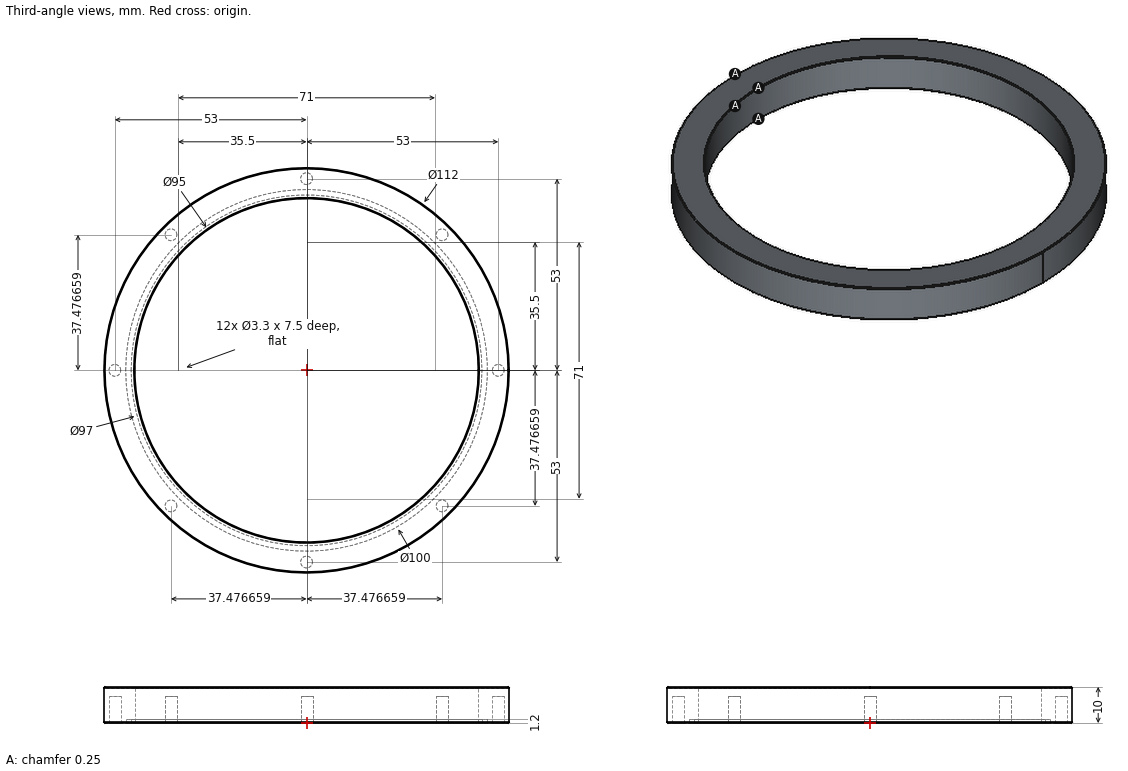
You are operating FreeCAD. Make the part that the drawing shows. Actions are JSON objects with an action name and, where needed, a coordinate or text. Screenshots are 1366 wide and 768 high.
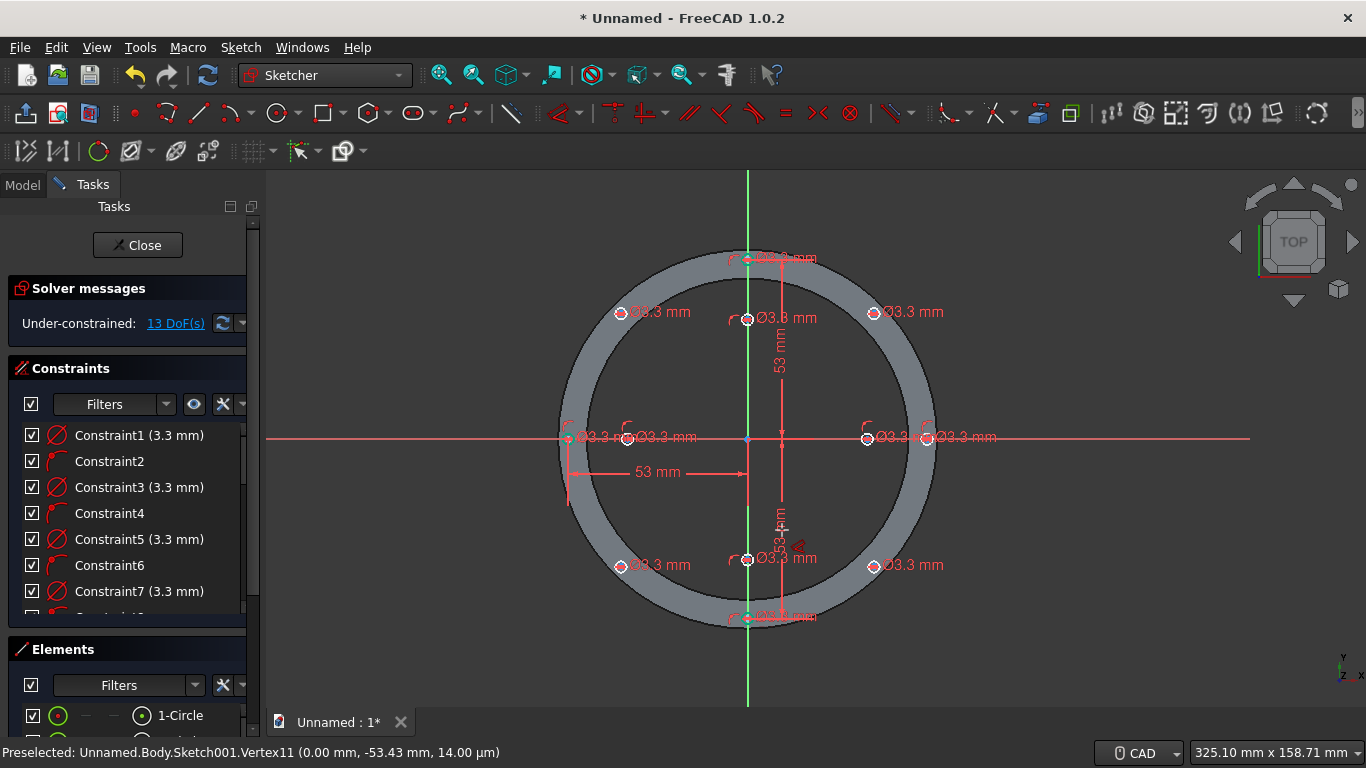
{"action": "left_click", "coordinate": [927, 439]}
{"action": "left_click", "coordinate": [837, 473]}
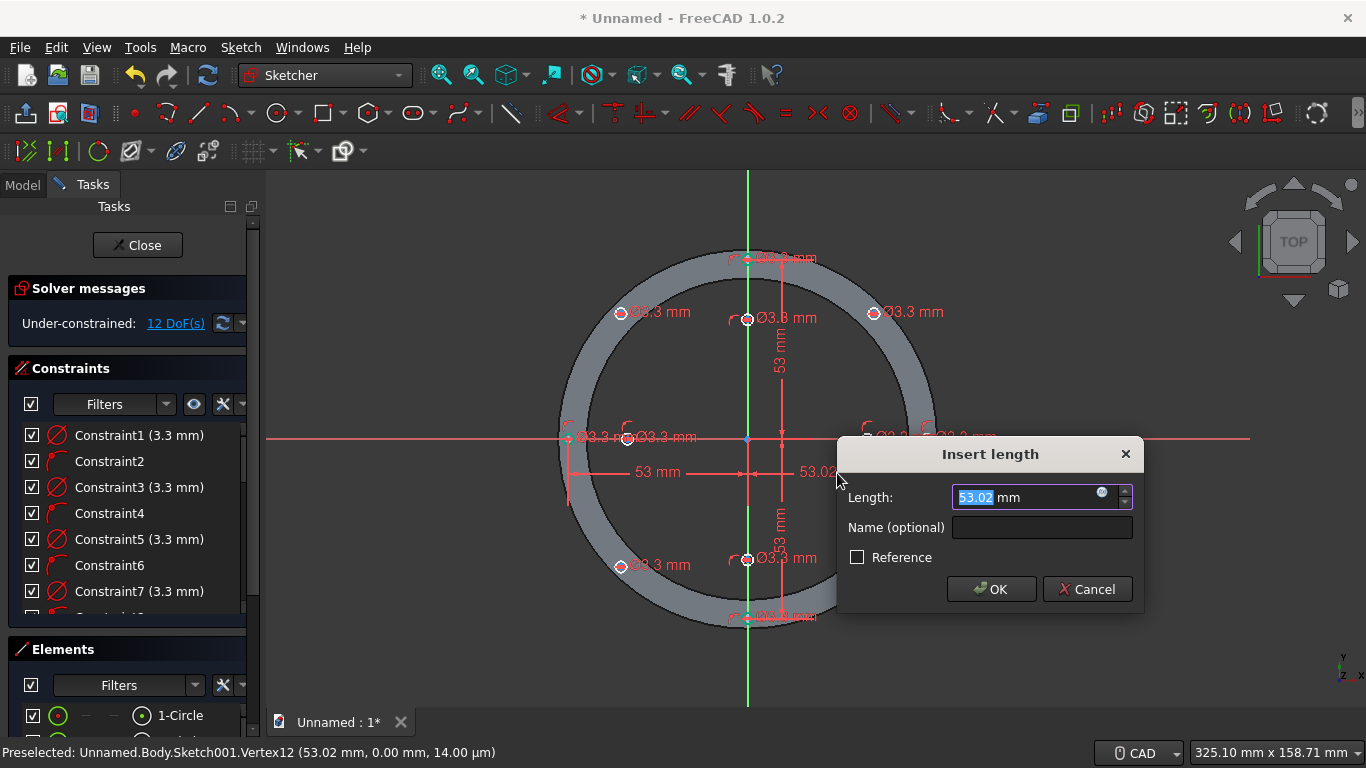
{"action": "type", "text": "53"}
{"action": "key", "text": "Return"}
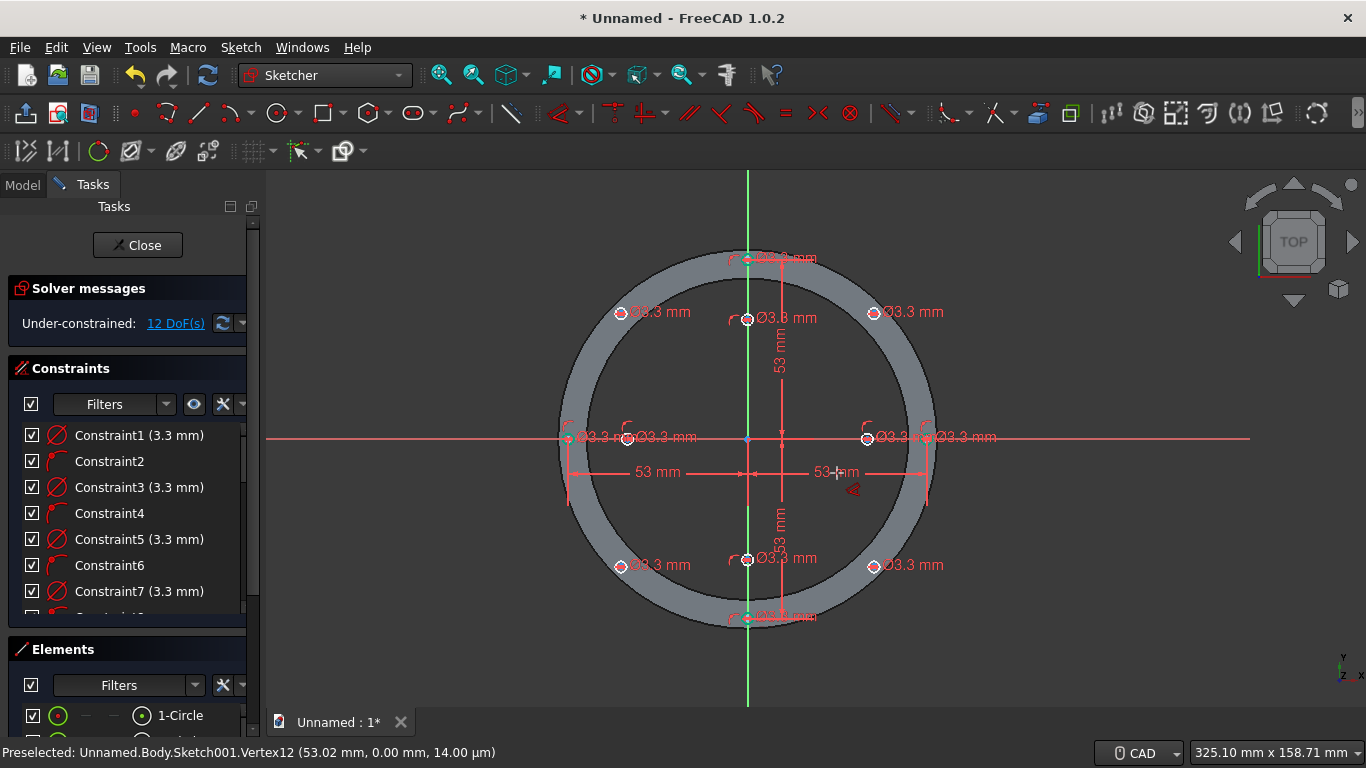
{"action": "left_click", "coordinate": [748, 320]}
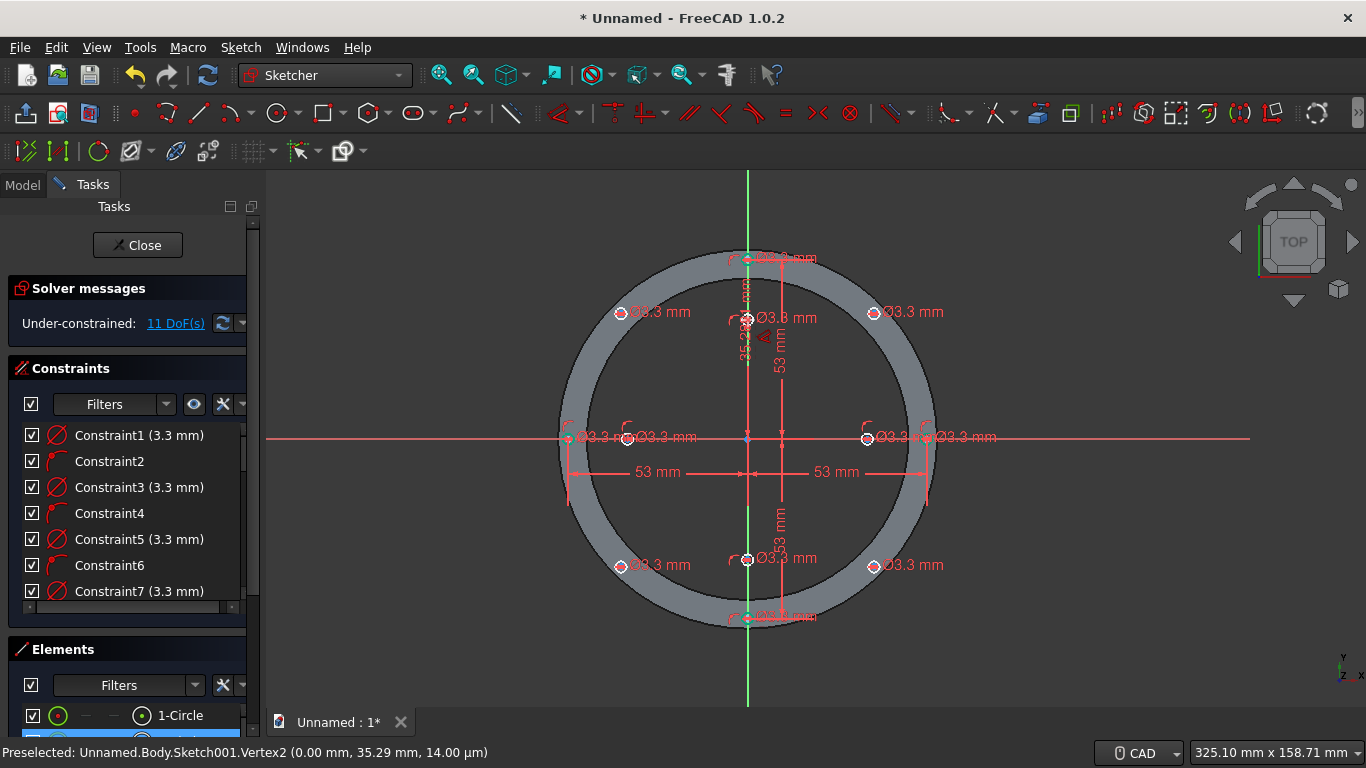
{"action": "left_click", "coordinate": [748, 560]}
{"action": "left_click", "coordinate": [782, 385]}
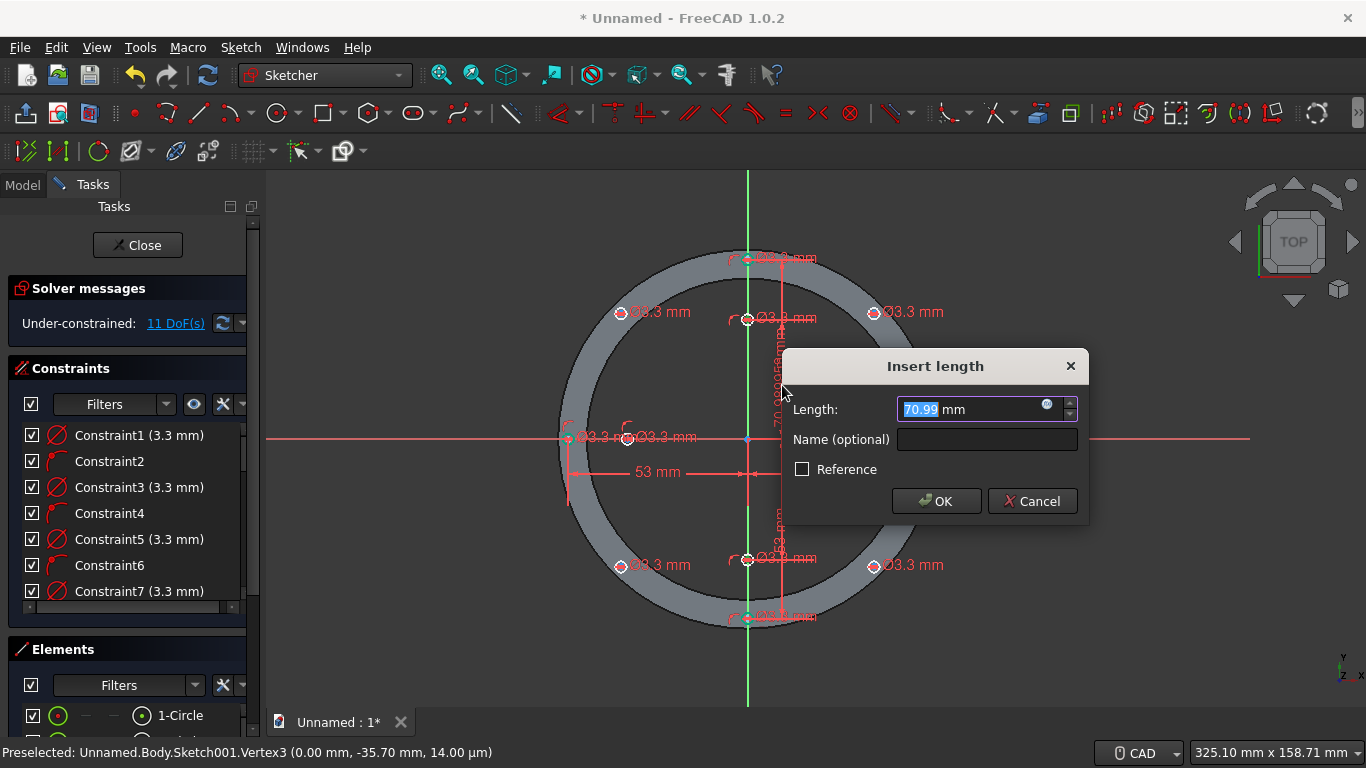
{"action": "type", "text": "71"}
{"action": "key", "text": "Return"}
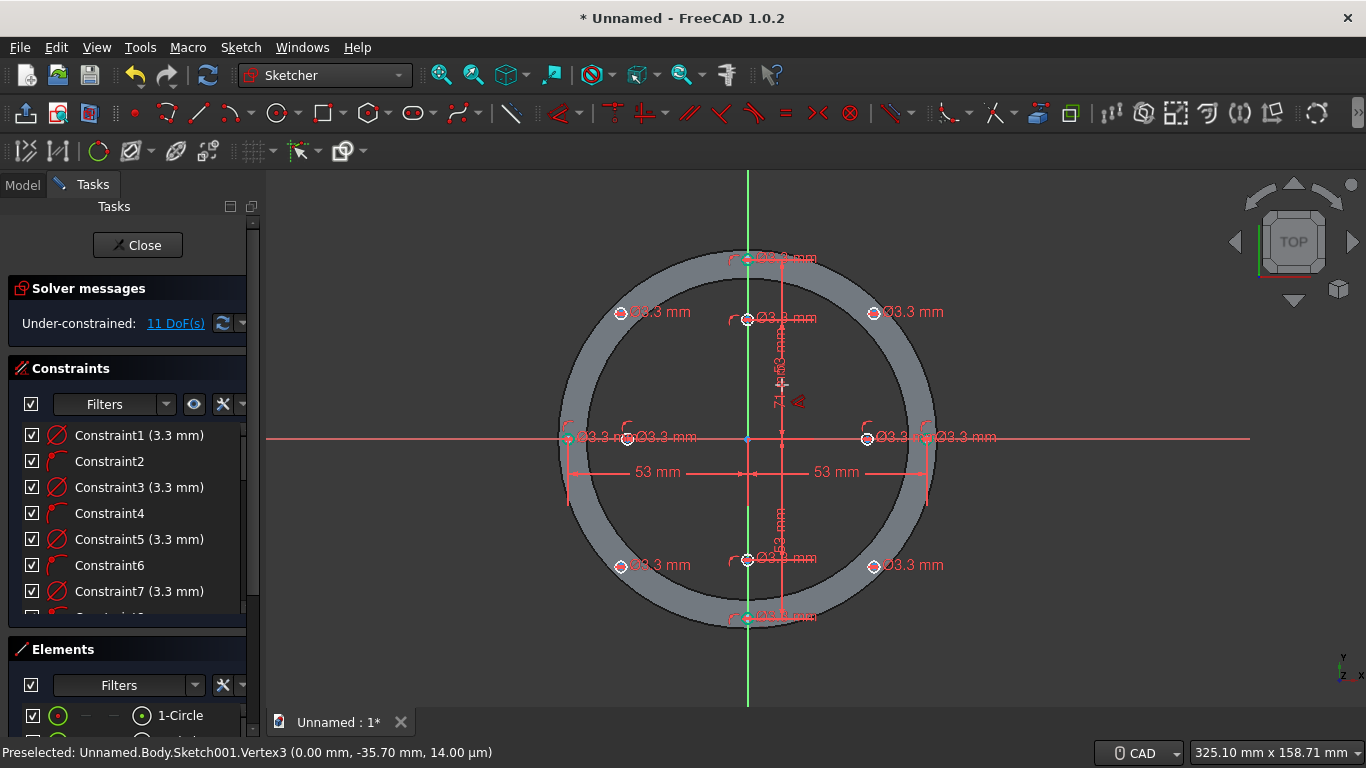
{"action": "left_click", "coordinate": [627, 439]}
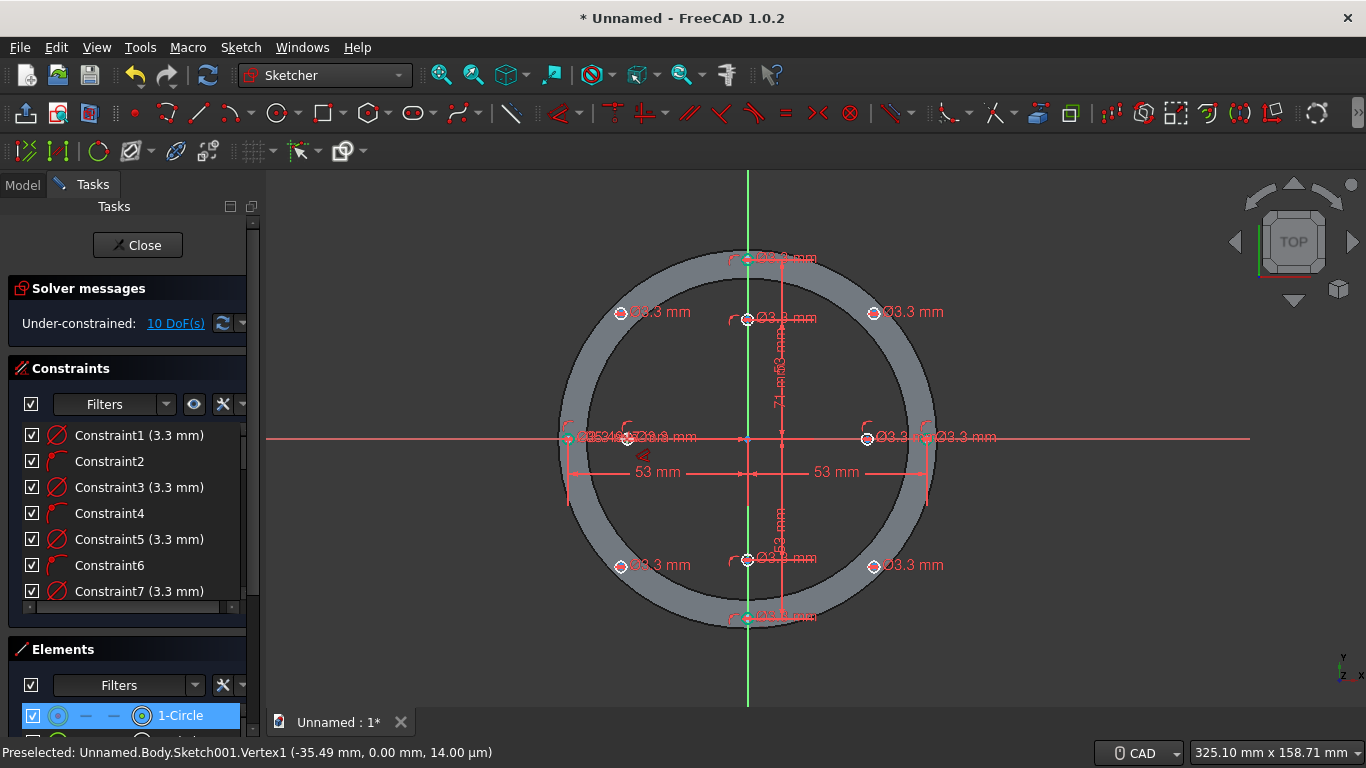
{"action": "left_click", "coordinate": [867, 439]}
{"action": "left_click", "coordinate": [692, 405]}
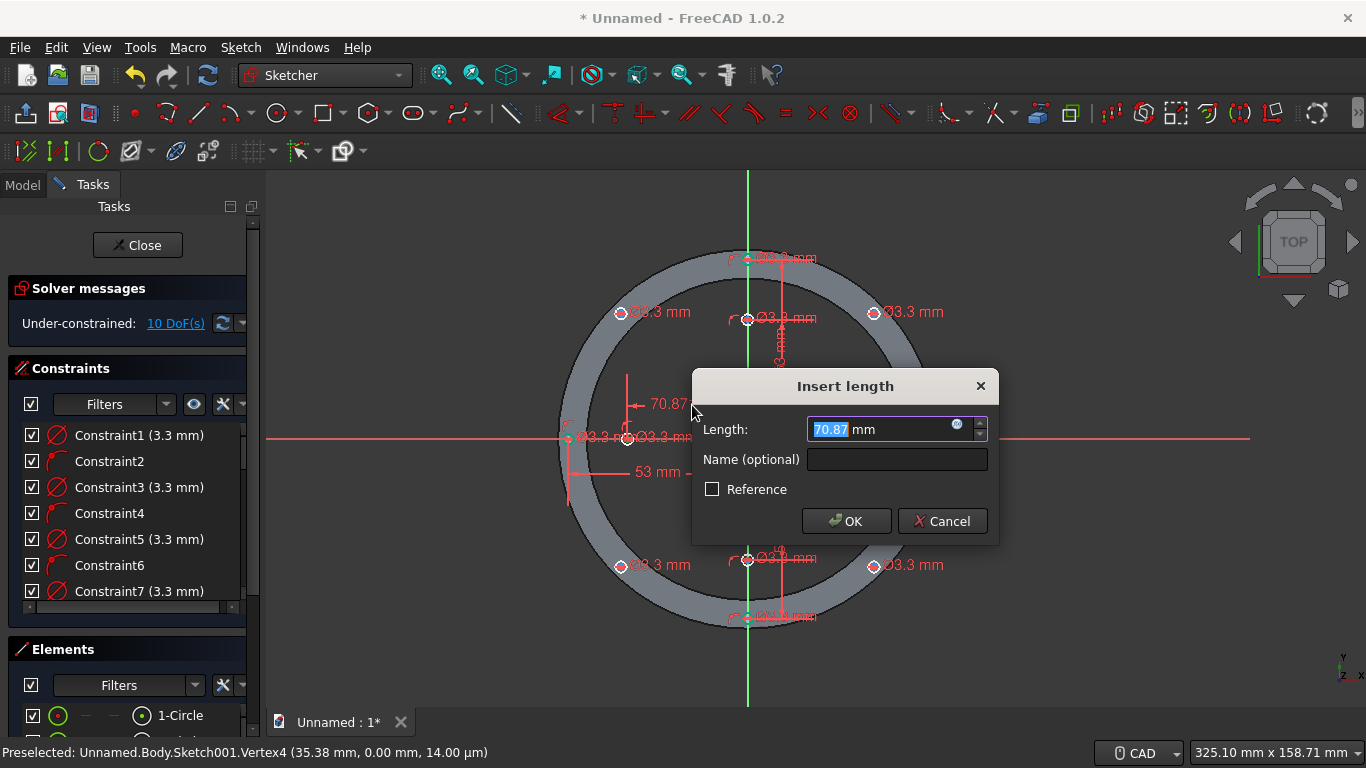
{"action": "type", "text": "71"}
{"action": "key", "text": "Return"}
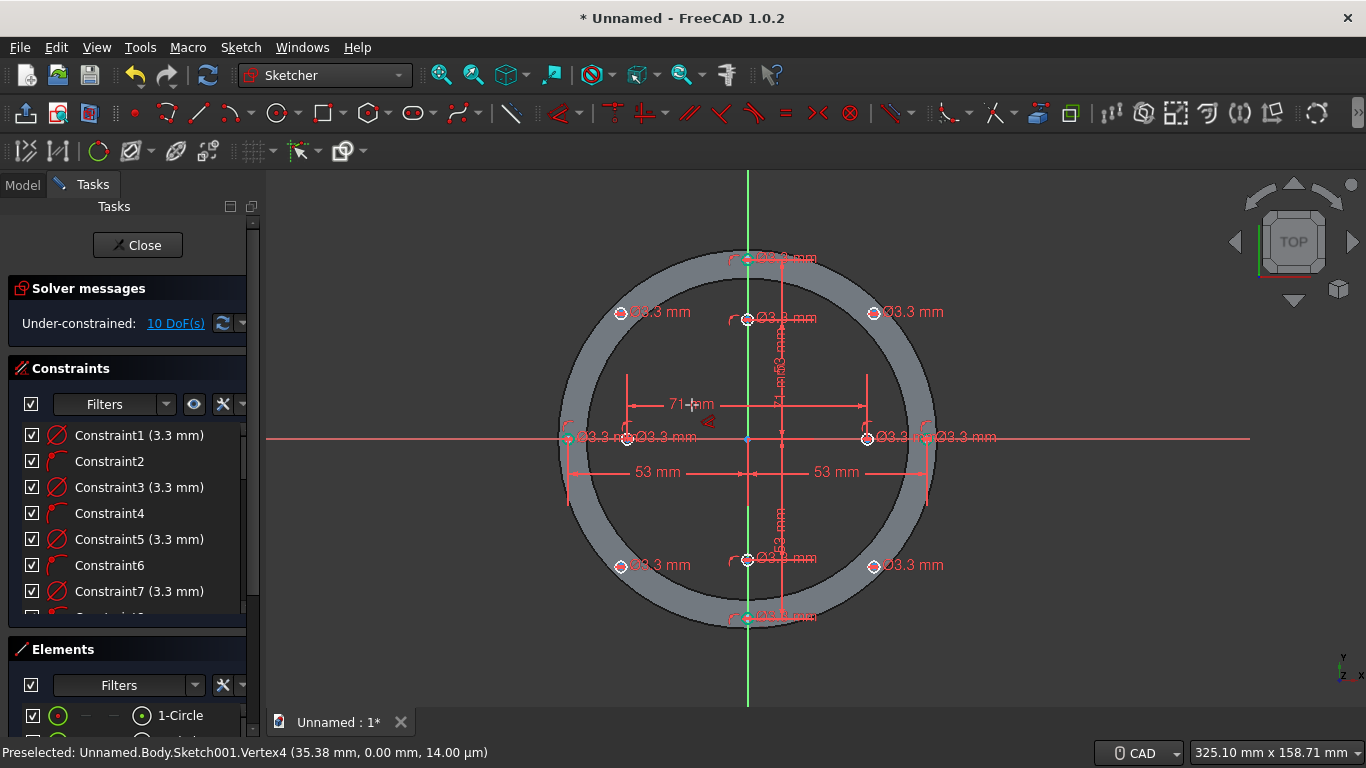
{"action": "left_click", "coordinate": [627, 439]}
{"action": "left_click", "coordinate": [730, 473]}